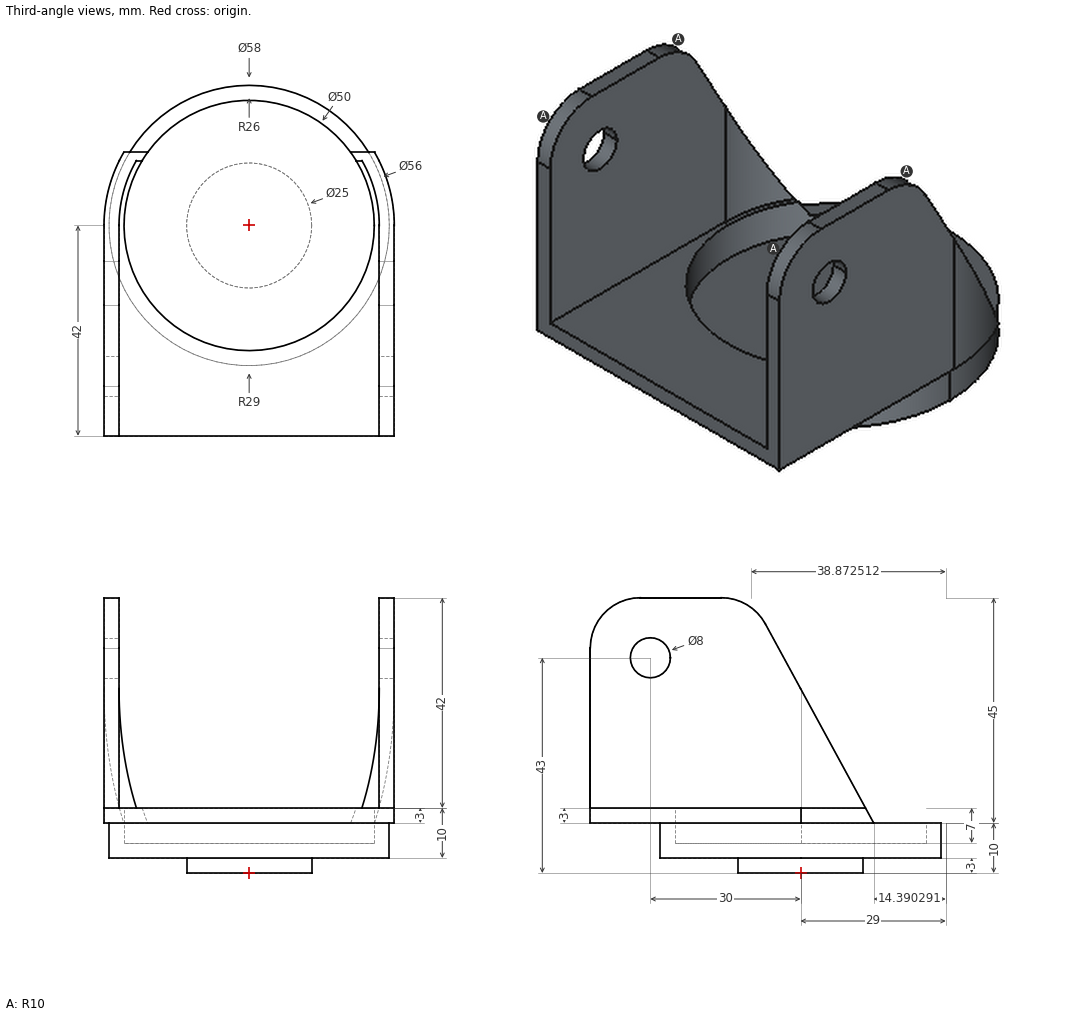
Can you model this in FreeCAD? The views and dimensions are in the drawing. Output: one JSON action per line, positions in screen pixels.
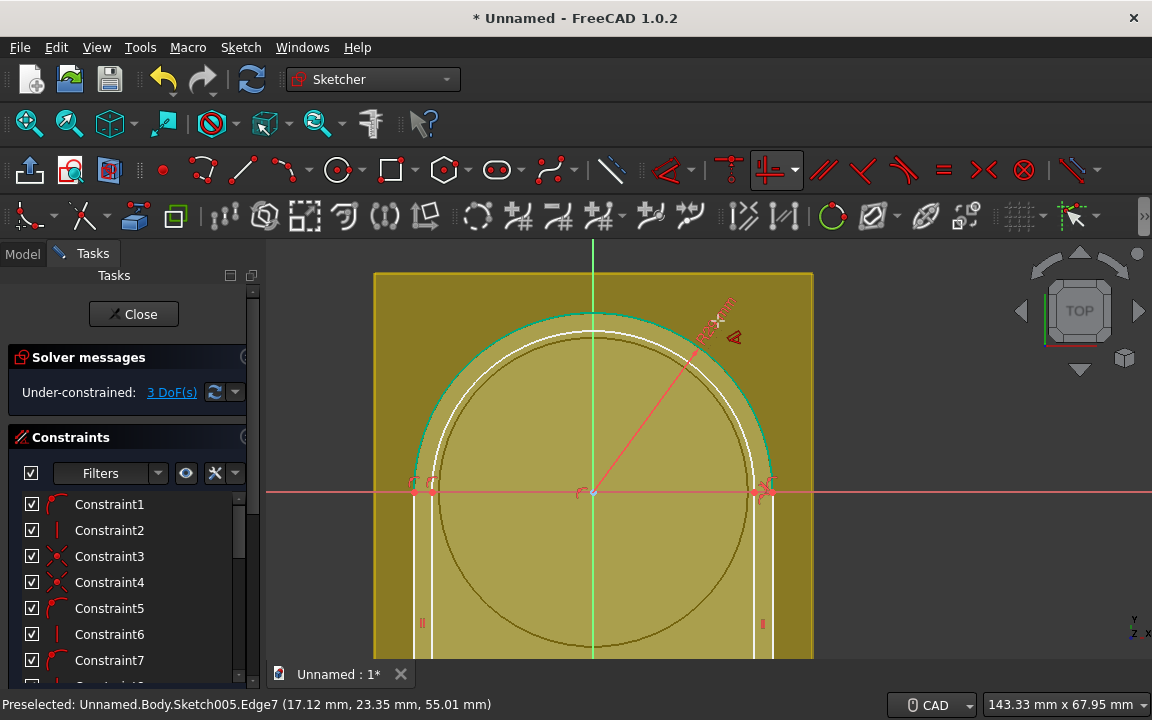
{"action": "left_click", "coordinate": [688, 362]}
{"action": "left_click", "coordinate": [768, 410]}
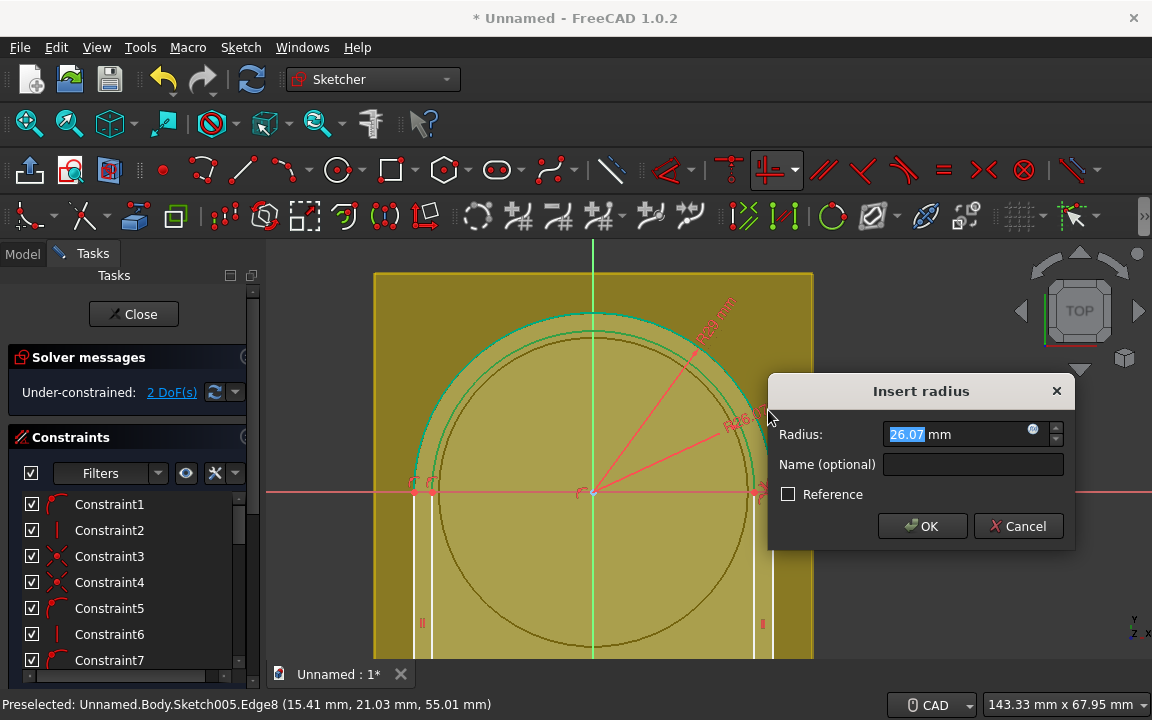
{"action": "type", "text": "26"}
{"action": "key", "text": "Return"}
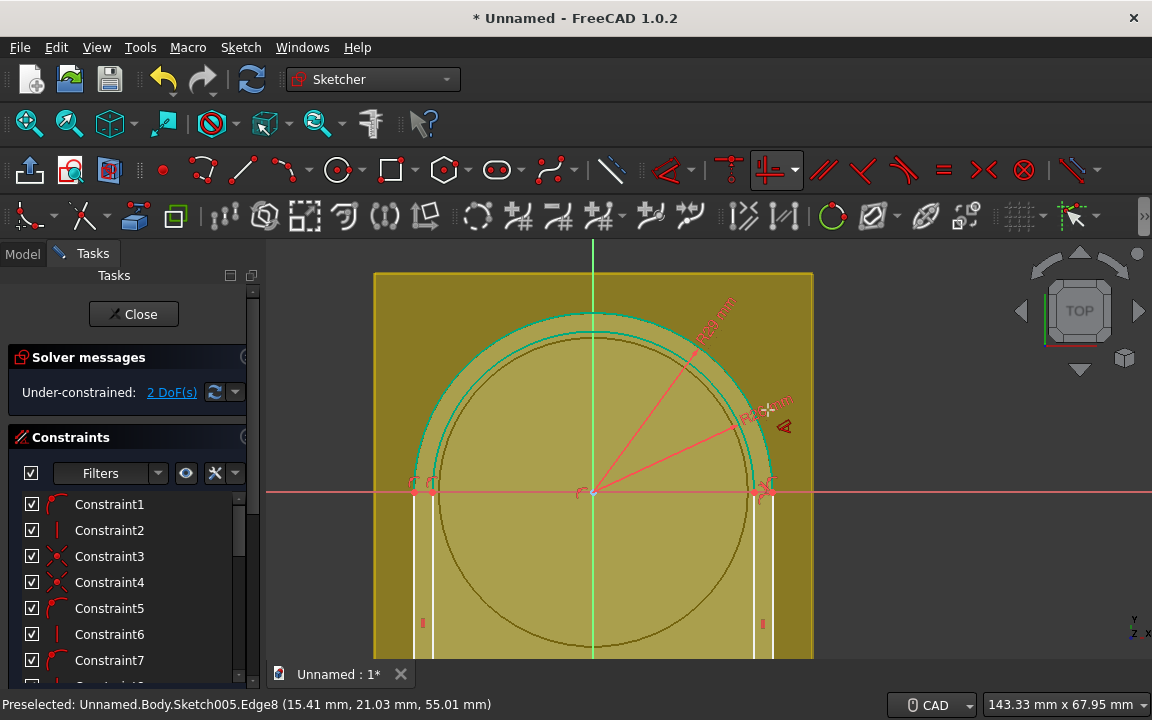
{"action": "left_click", "coordinate": [754, 571]}
{"action": "left_click", "coordinate": [788, 562]}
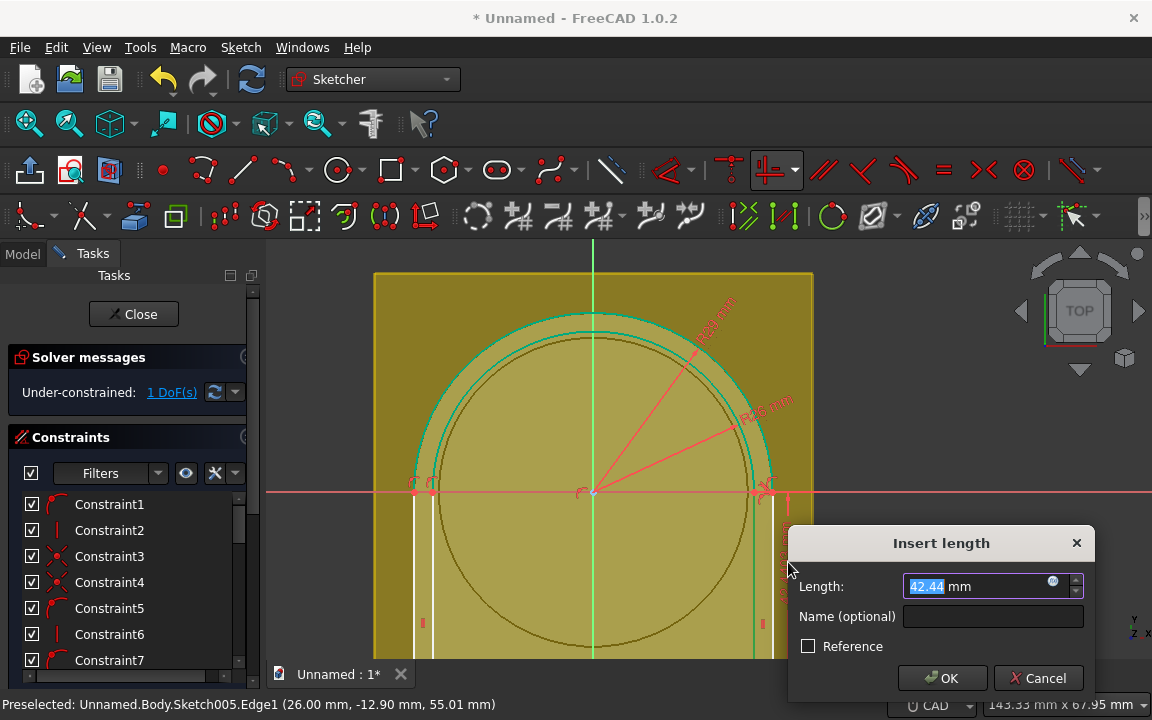
{"action": "type", "text": "42"}
{"action": "key", "text": "Return"}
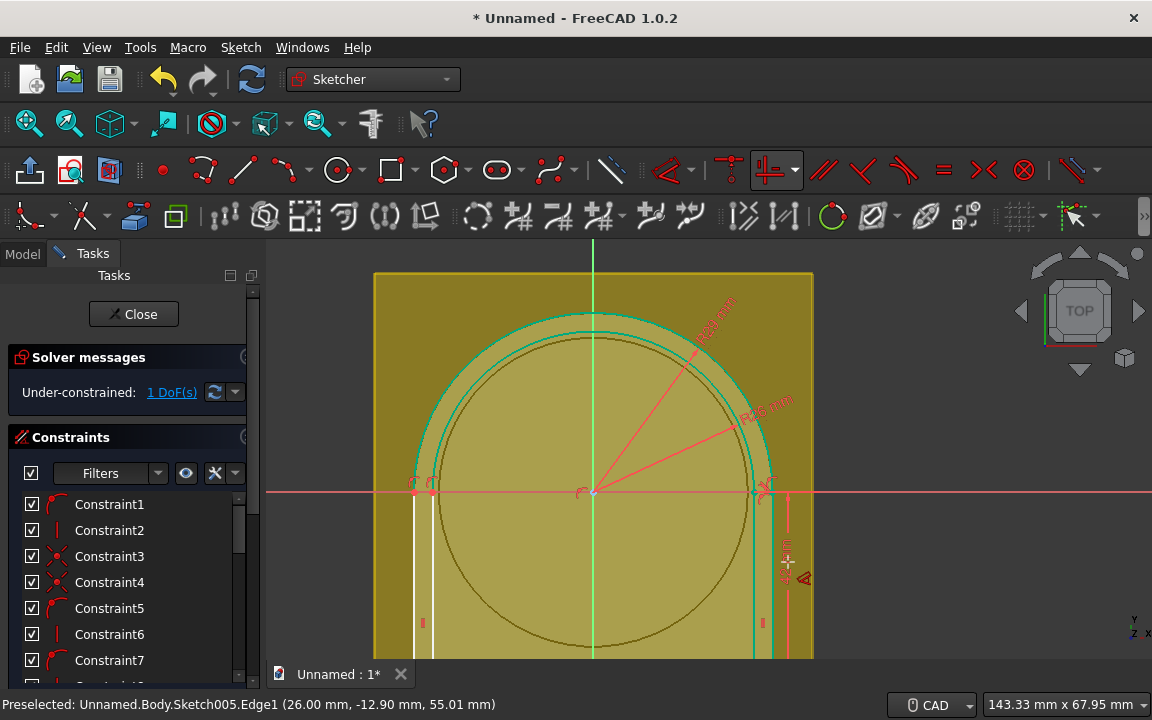
{"action": "left_click", "coordinate": [414, 570]}
{"action": "left_click", "coordinate": [380, 562]}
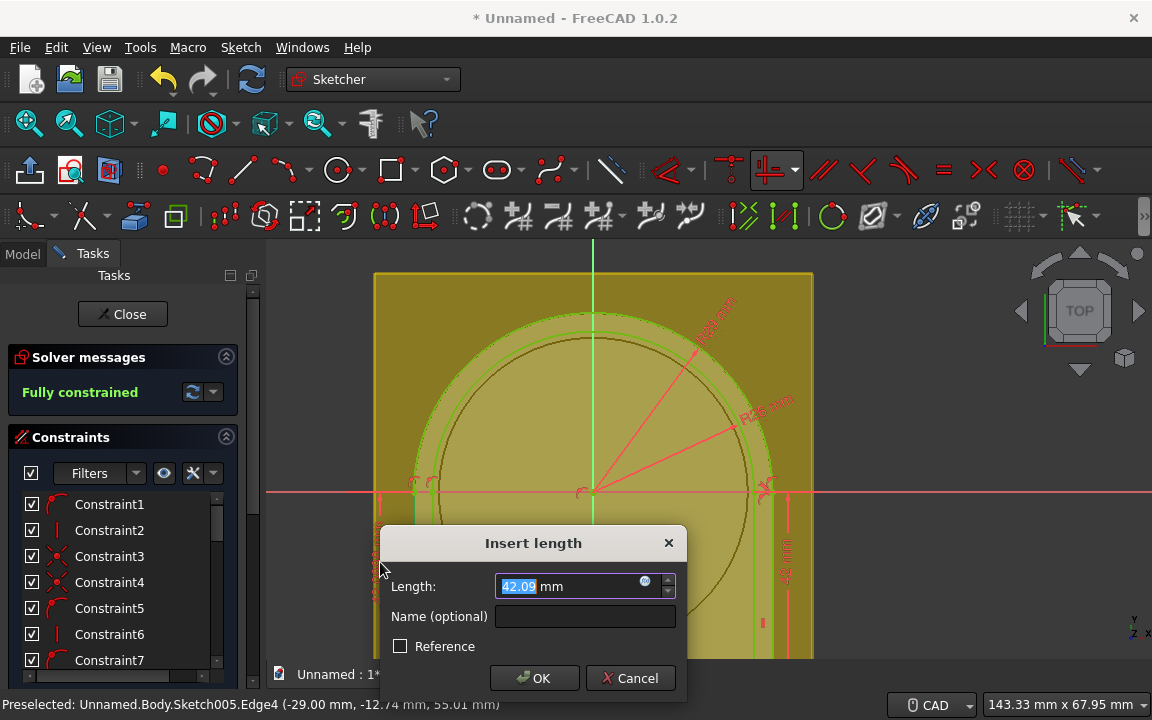
{"action": "type", "text": "42"}
{"action": "key", "text": "Return"}
{"action": "key", "text": "Escape"}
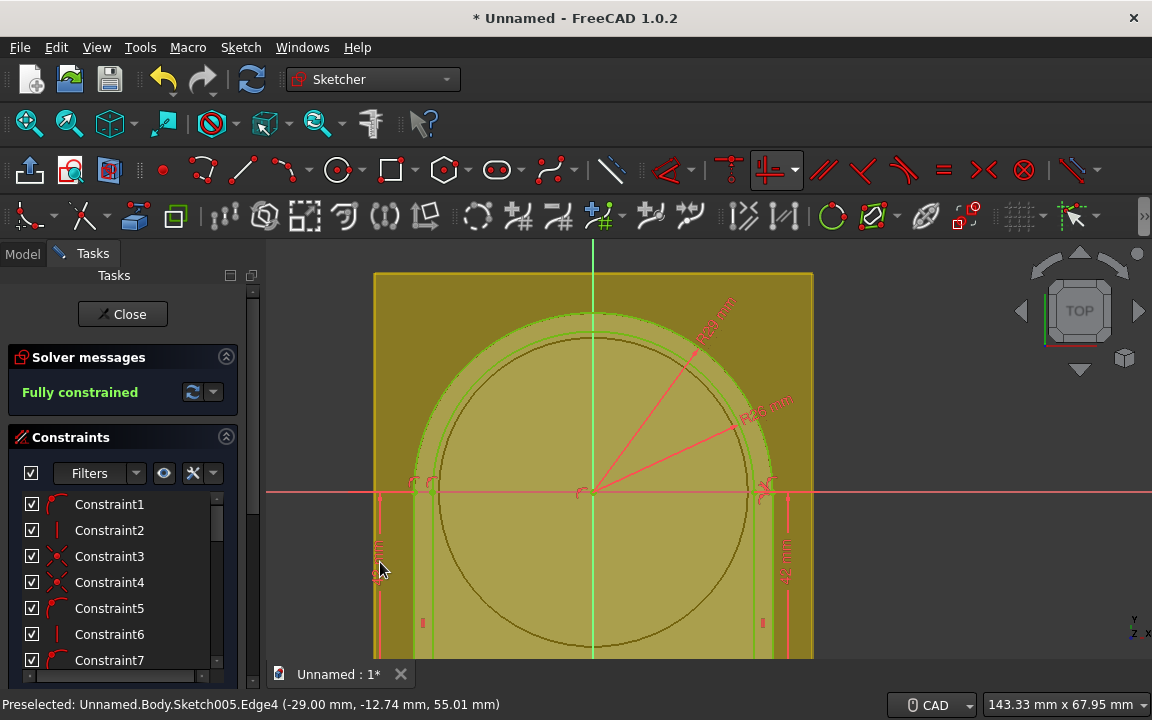
{"action": "left_click", "coordinate": [123, 314]}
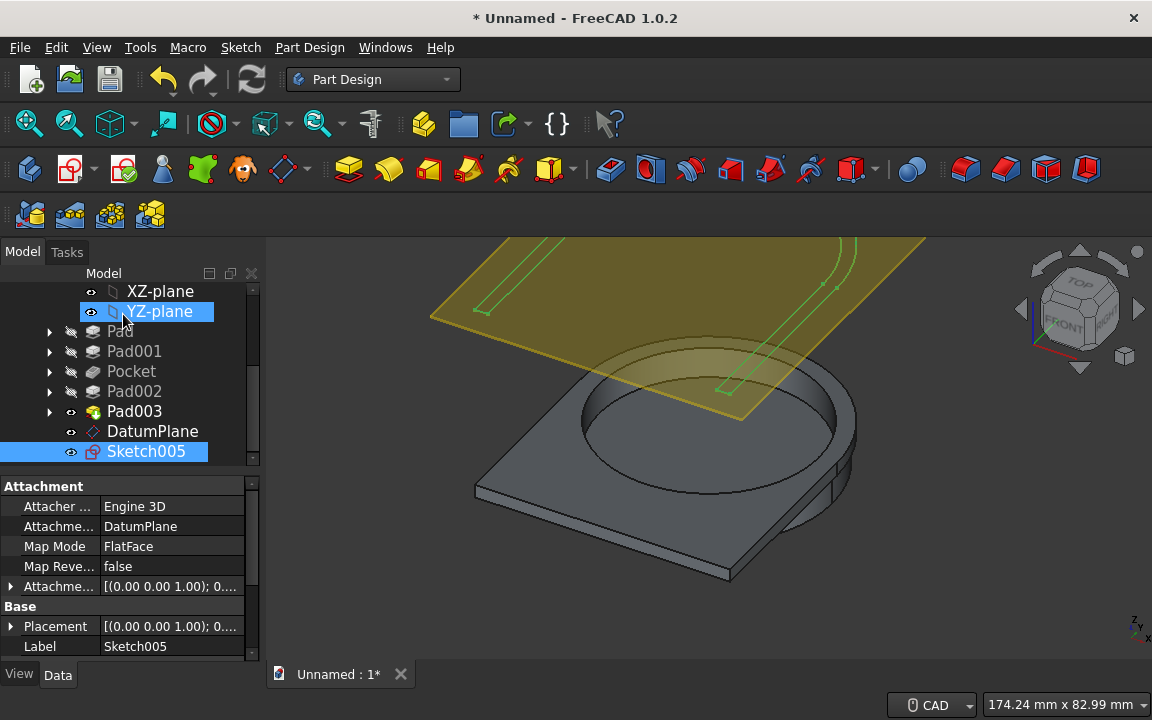
{"action": "left_click", "coordinate": [350, 170]}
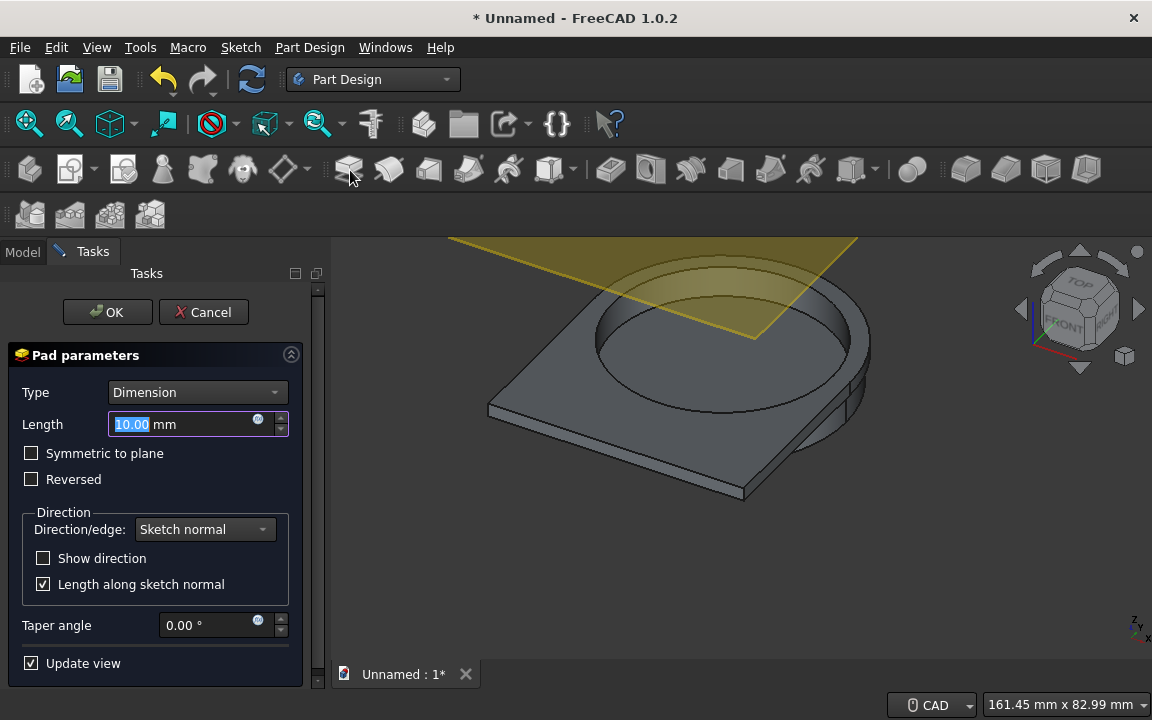
{"action": "type", "text": "42"}
{"action": "key", "text": "Tab"}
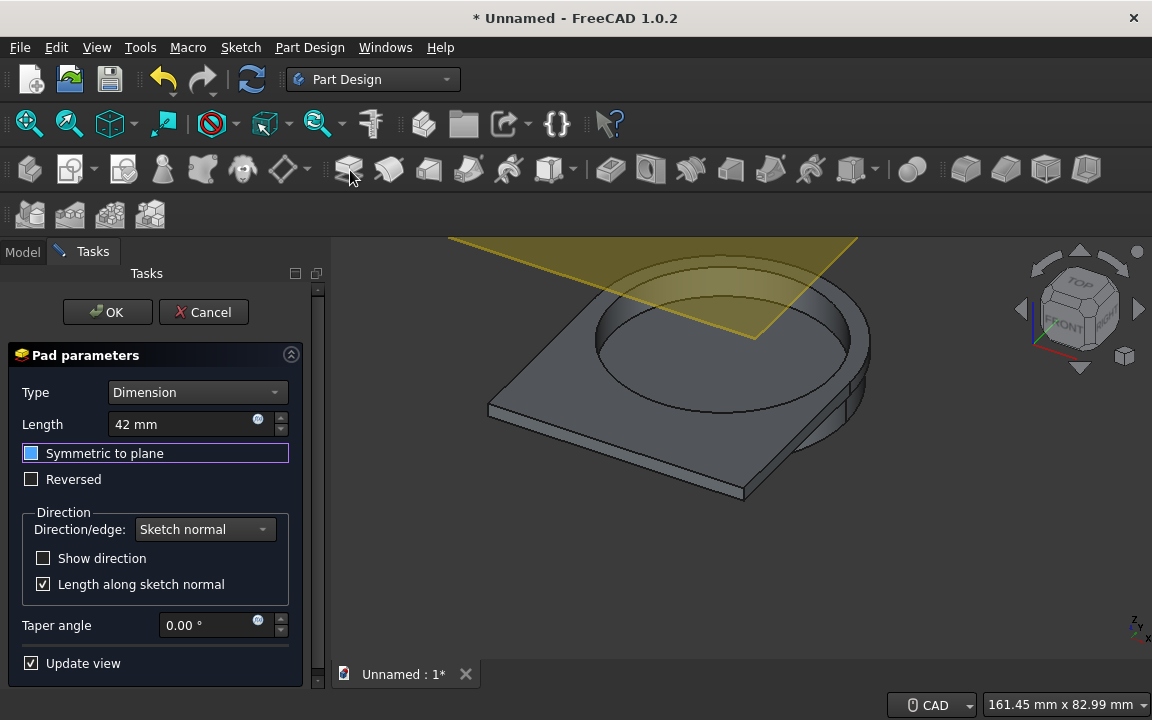
{"action": "left_click", "coordinate": [30, 479]}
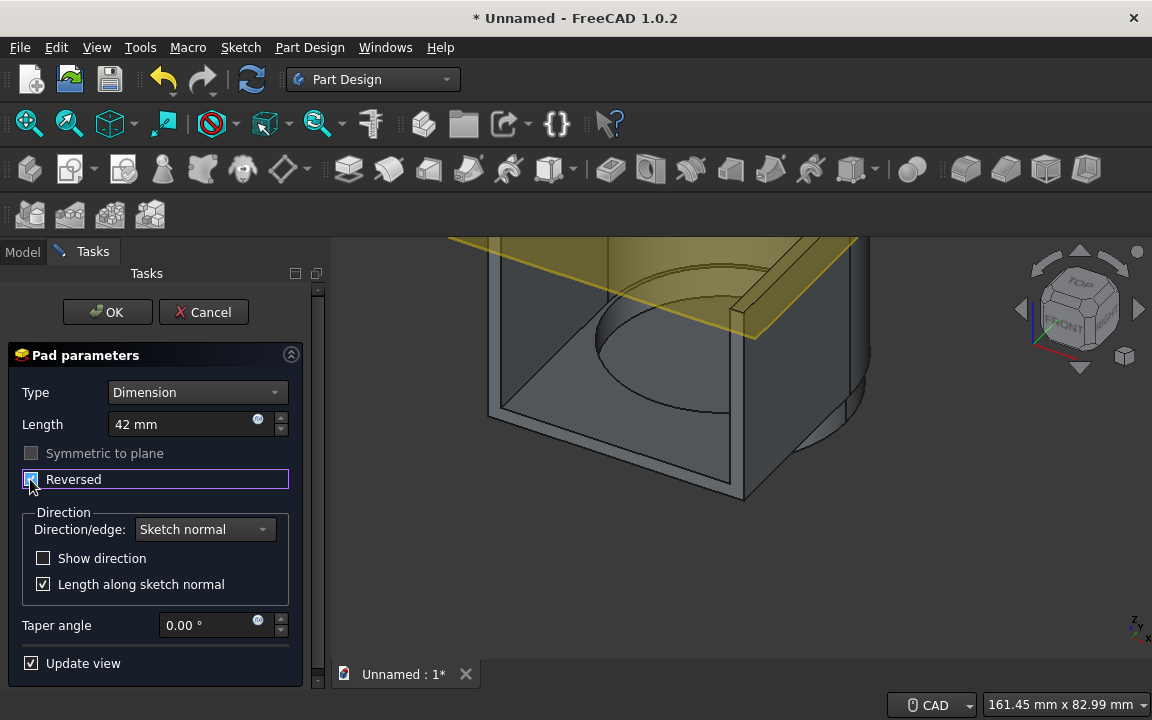
{"action": "left_click", "coordinate": [108, 312]}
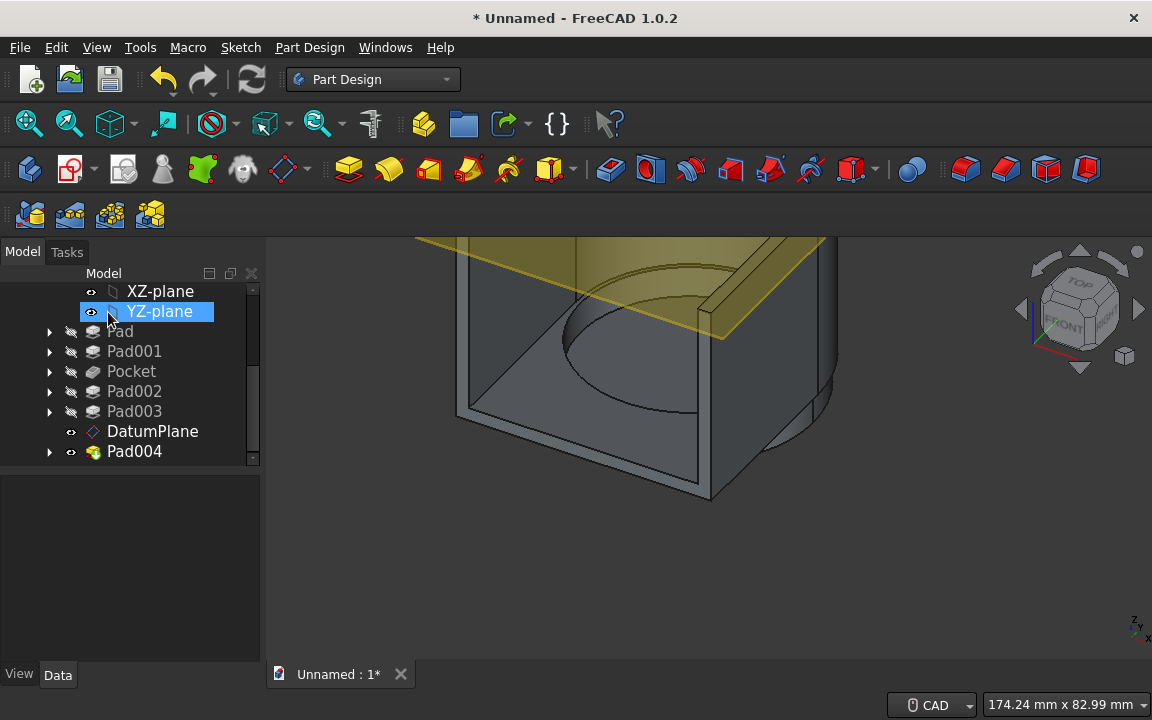
{"action": "left_click", "coordinate": [116, 432]}
{"action": "key", "text": "space"}